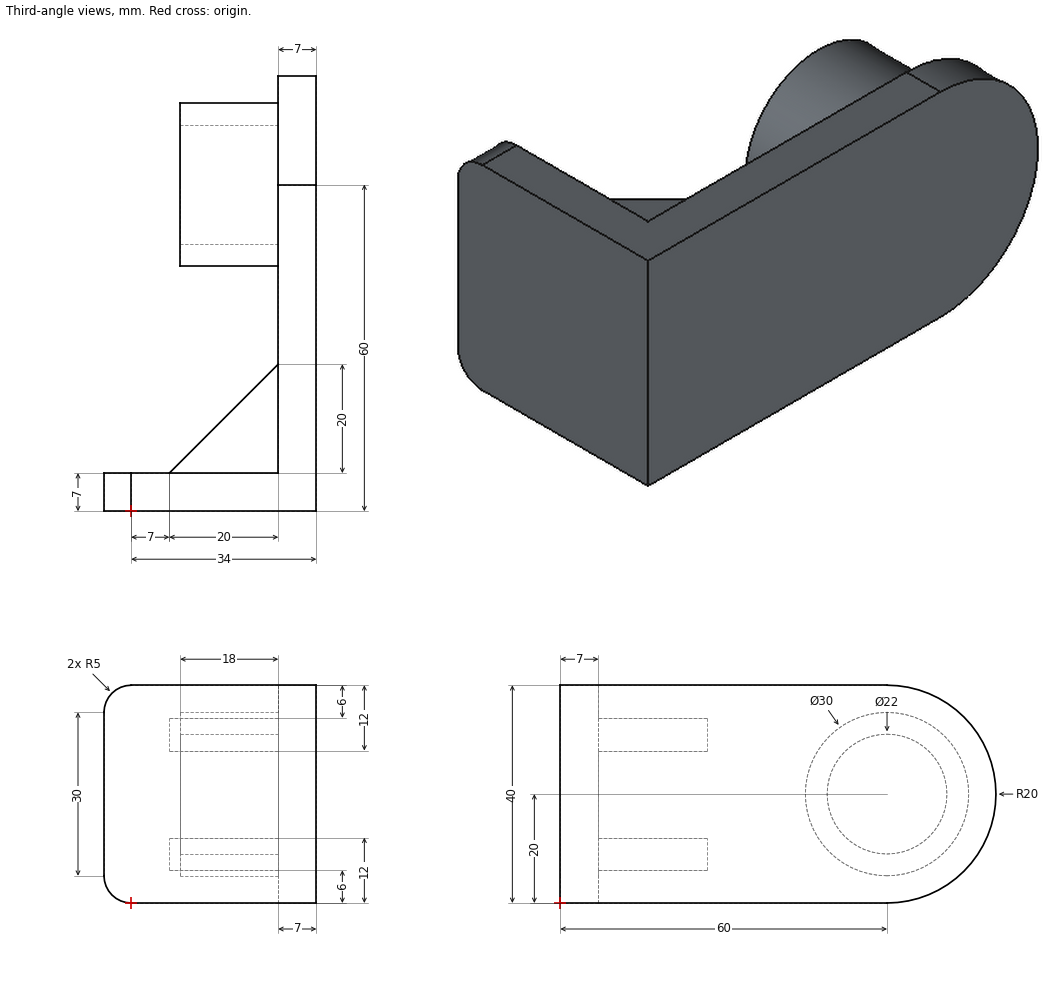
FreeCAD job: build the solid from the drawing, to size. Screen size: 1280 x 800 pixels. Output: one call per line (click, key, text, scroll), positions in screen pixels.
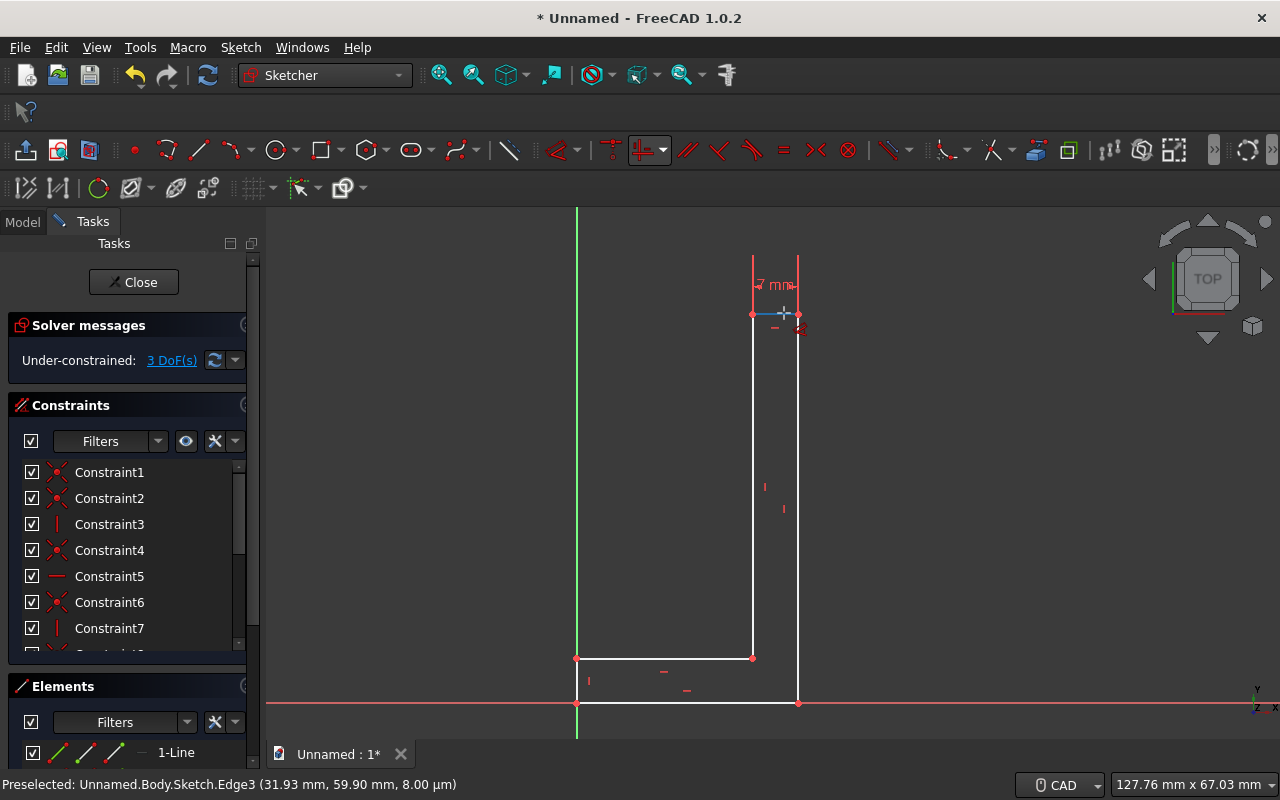
scroll(614, 607, up, 2)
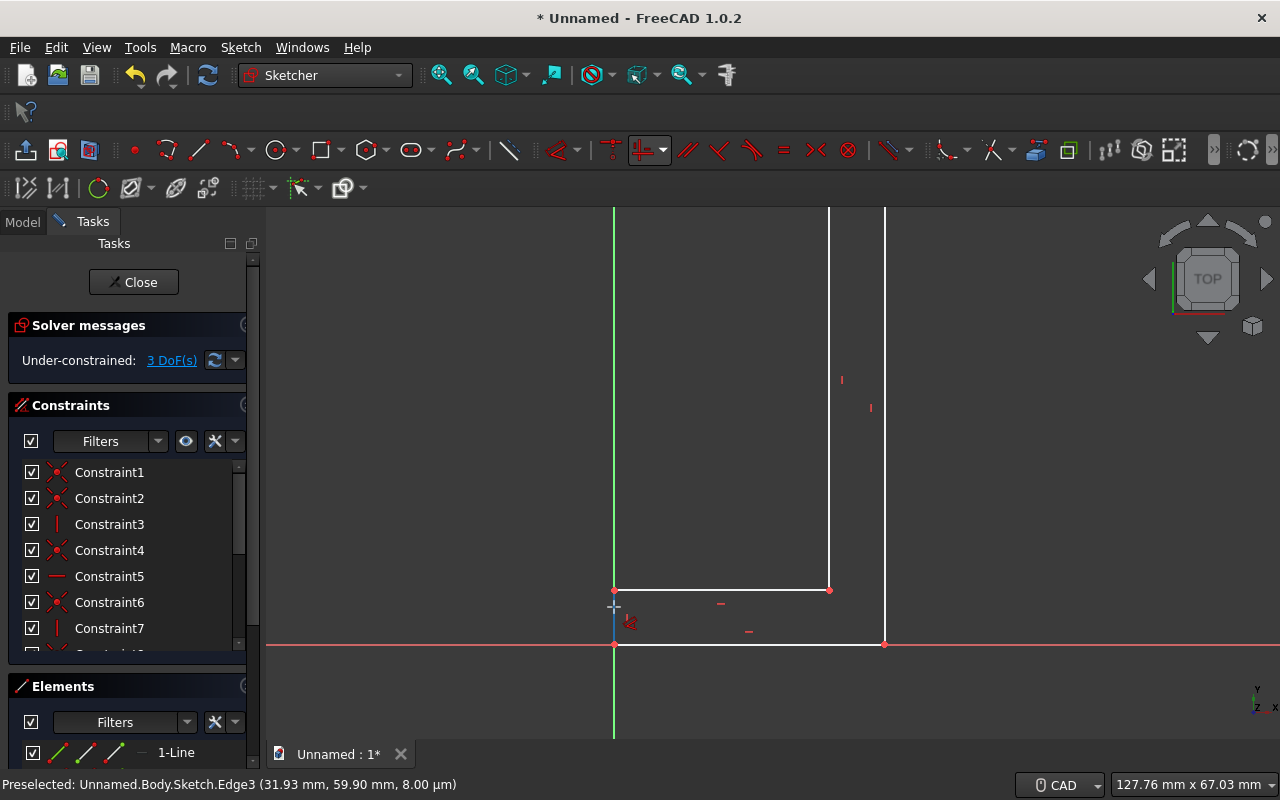
click(614, 607)
click(580, 618)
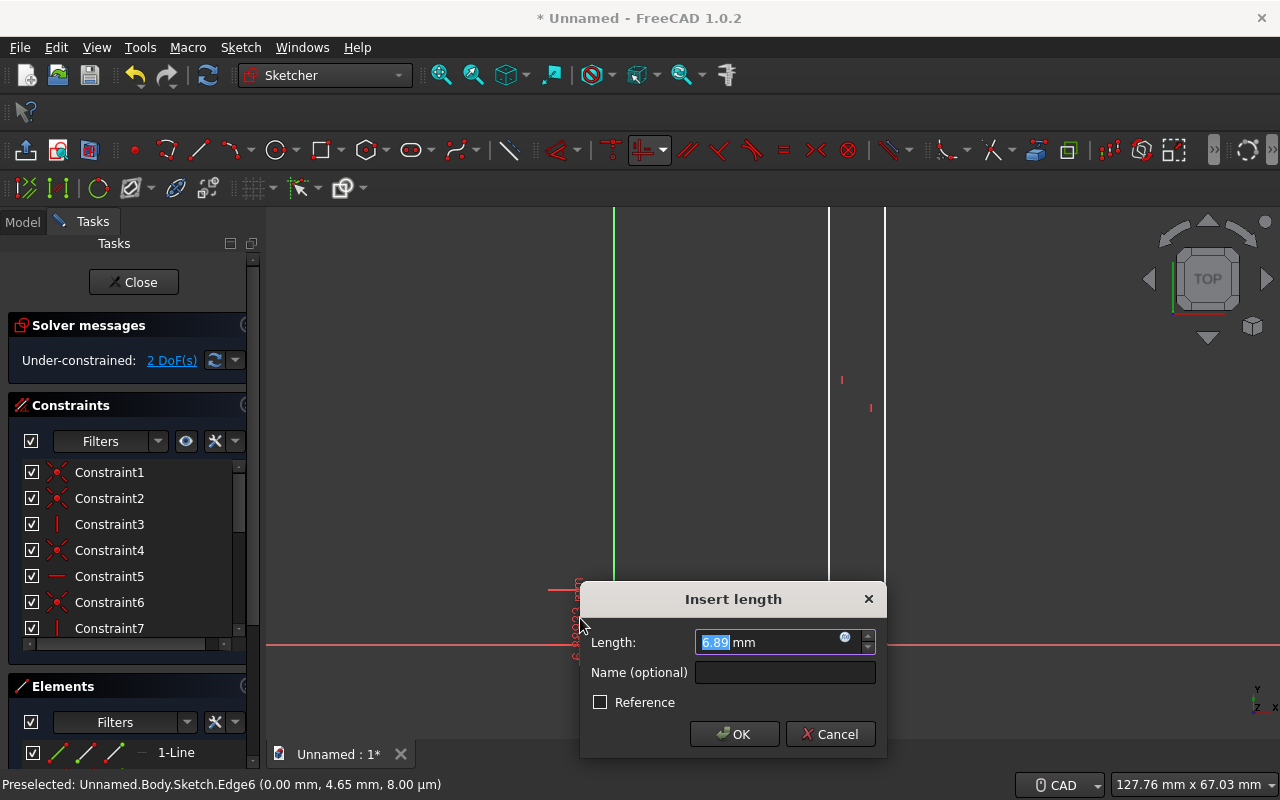
text(7)
key(Return)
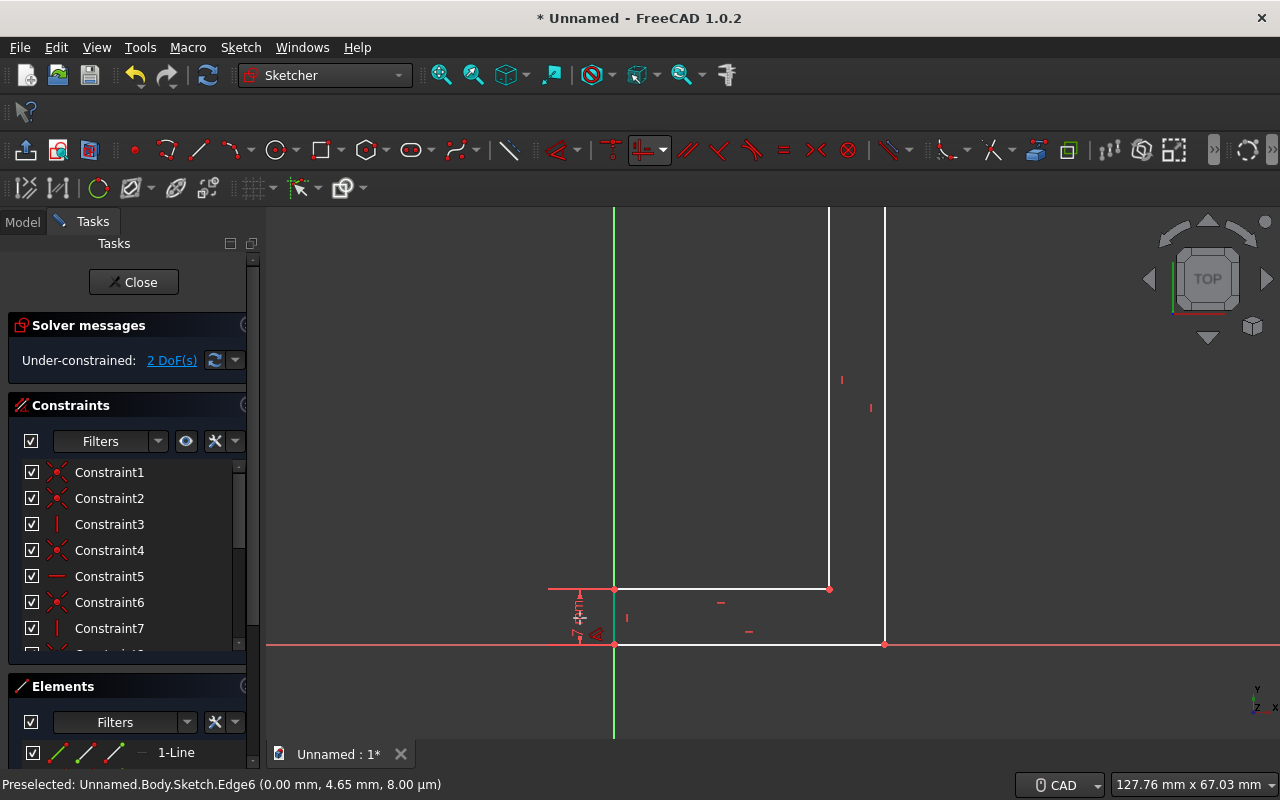
click(695, 645)
click(750, 679)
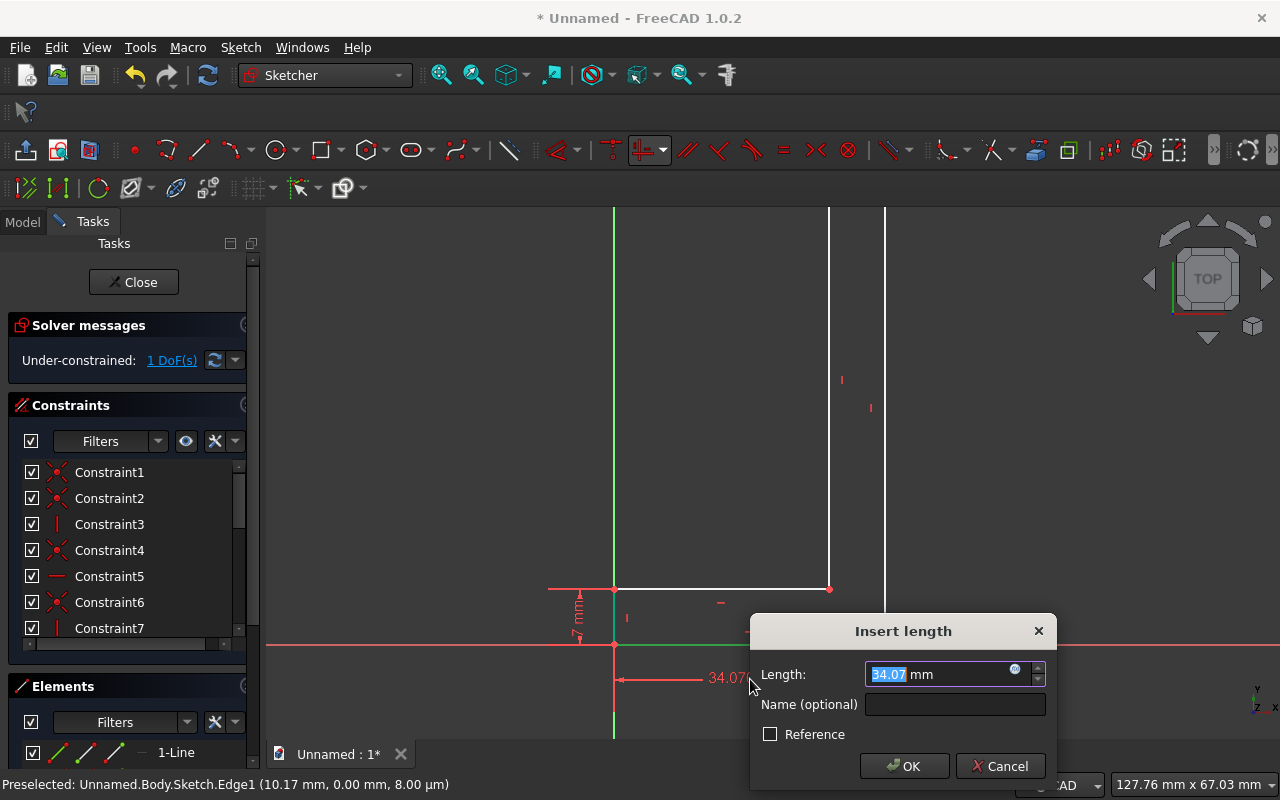
text(34)
key(Return)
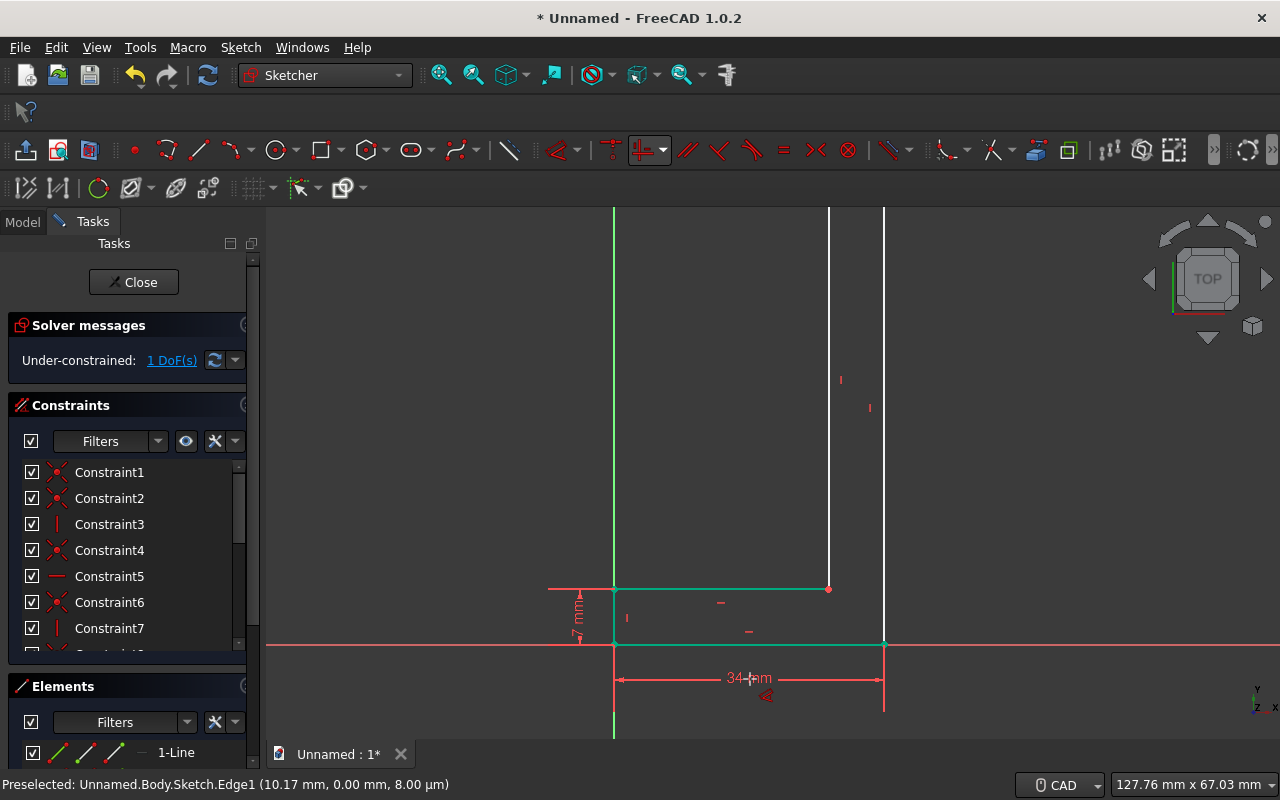
click(884, 502)
click(918, 440)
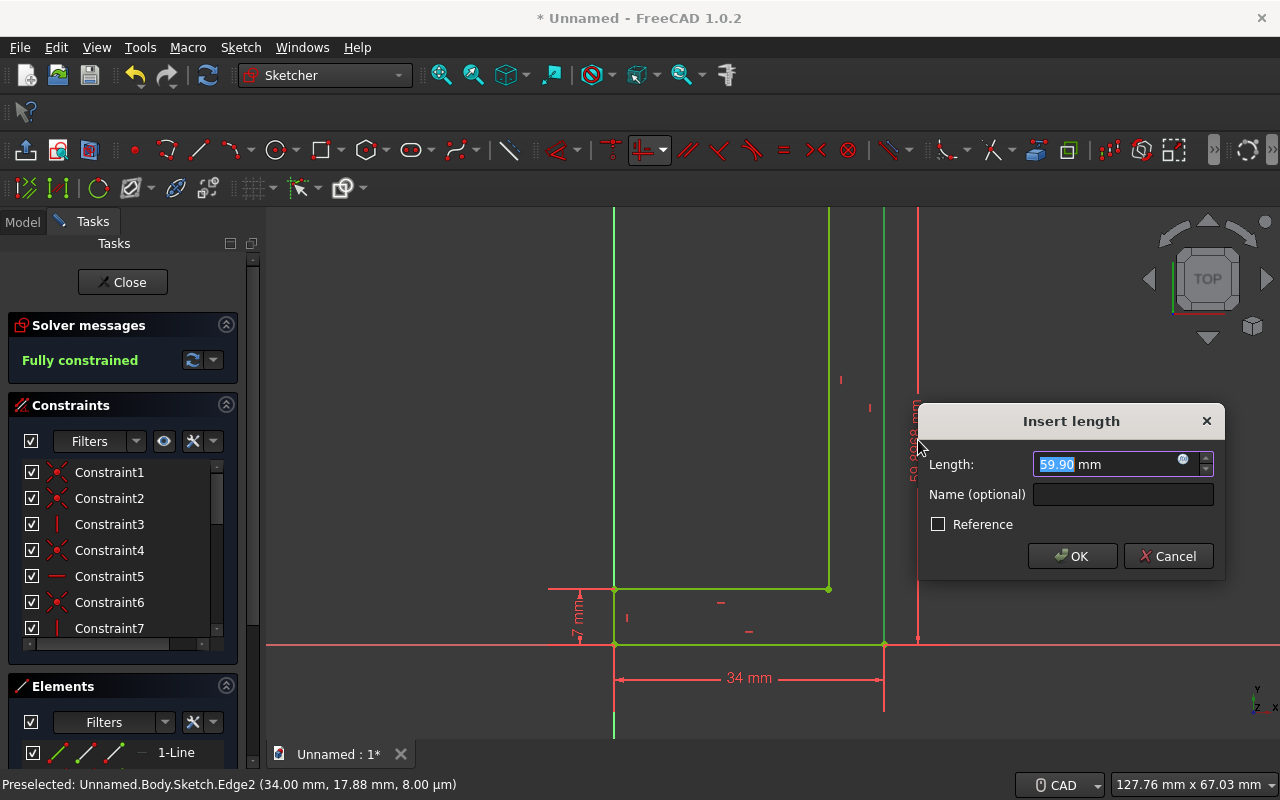
text(60)
key(Return)
key(Escape)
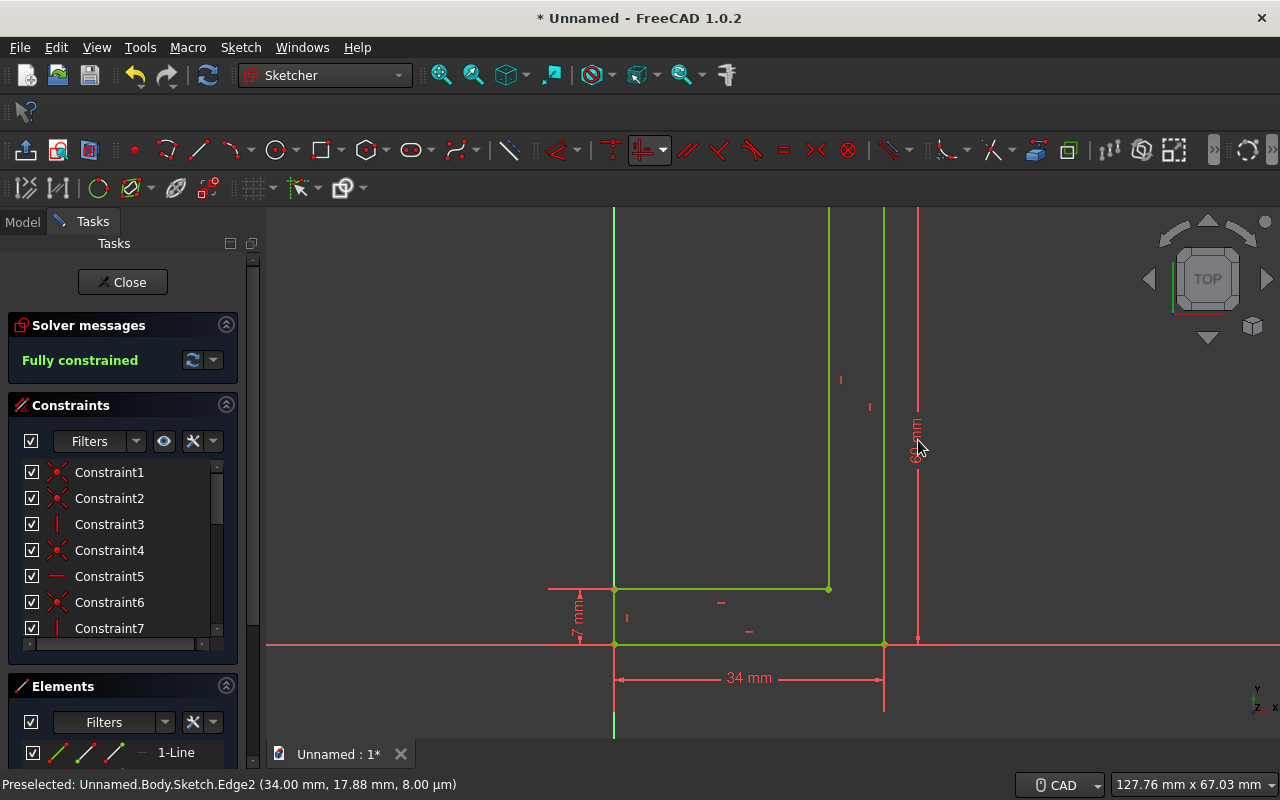
click(123, 282)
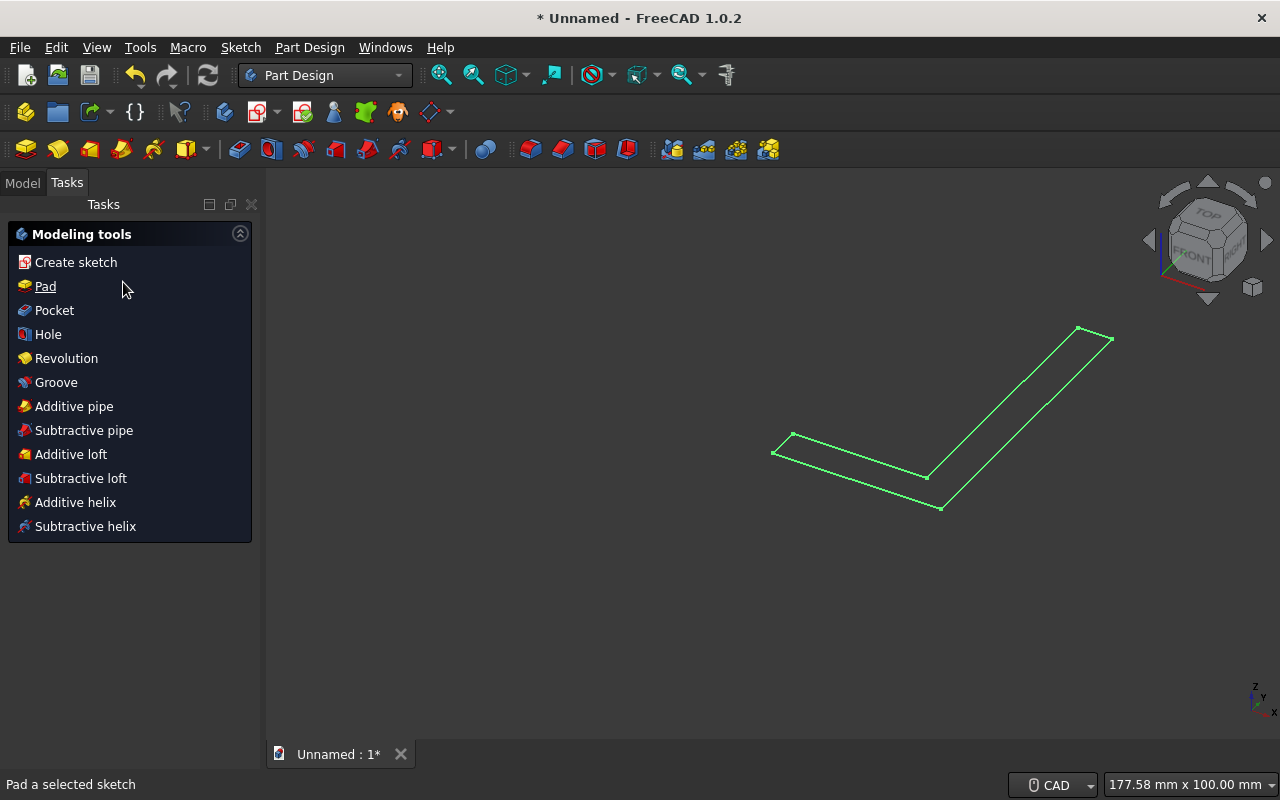
click(26, 150)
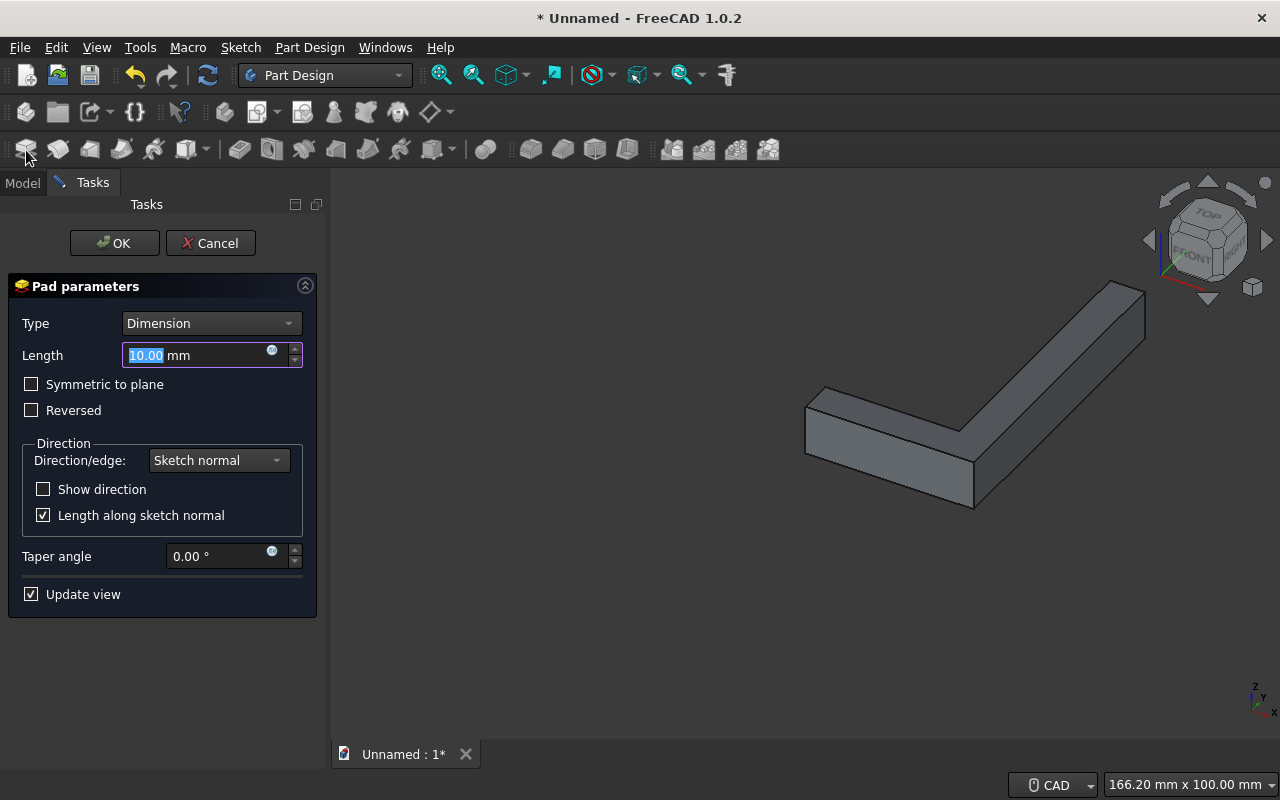
text(40)
key(Tab)